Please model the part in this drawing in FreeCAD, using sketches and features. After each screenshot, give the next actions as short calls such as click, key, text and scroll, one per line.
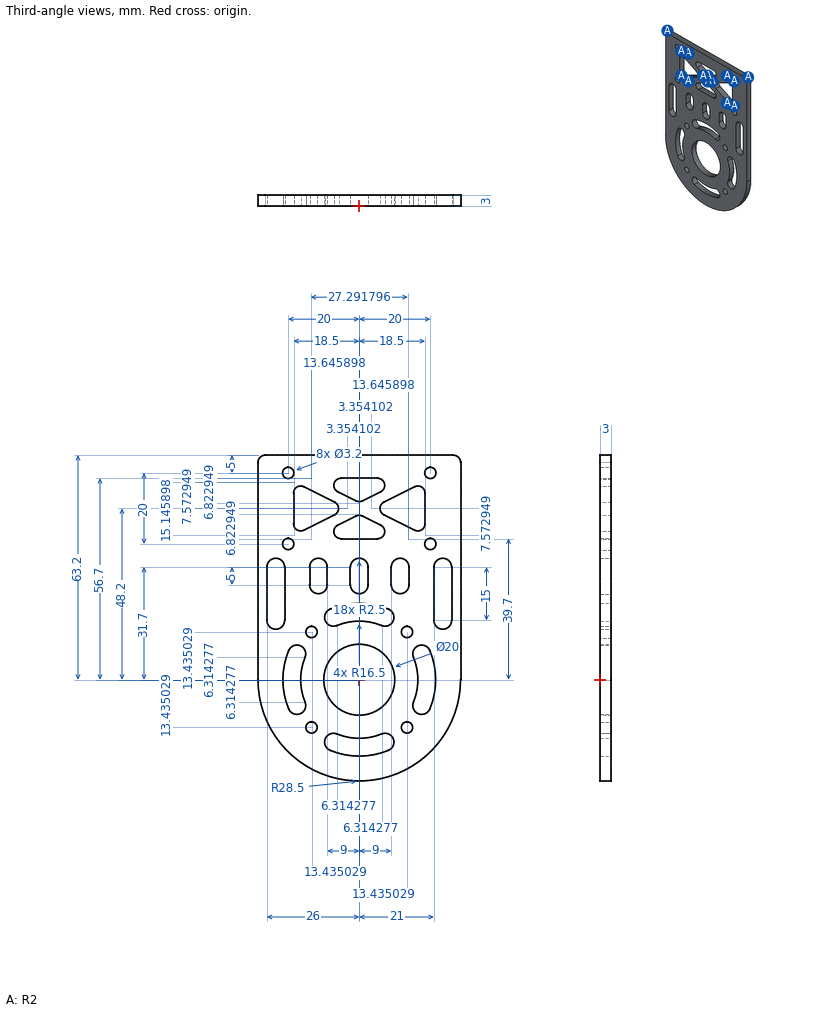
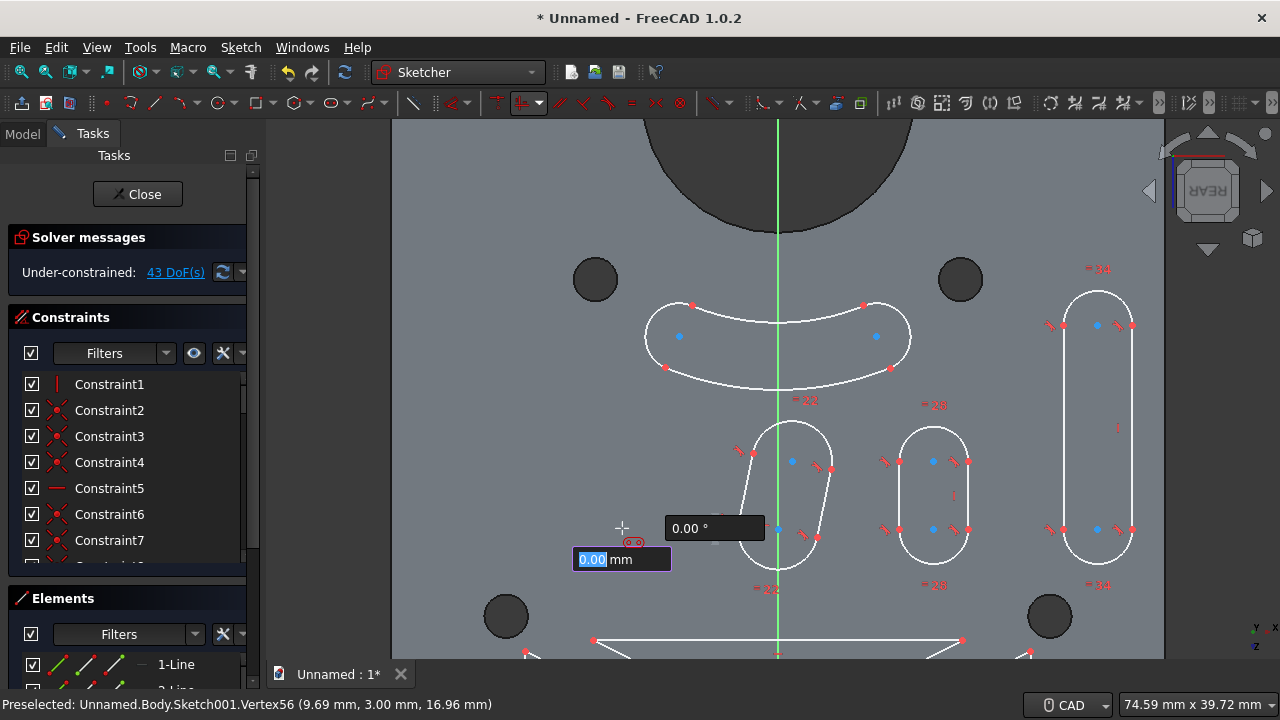
click(622, 460)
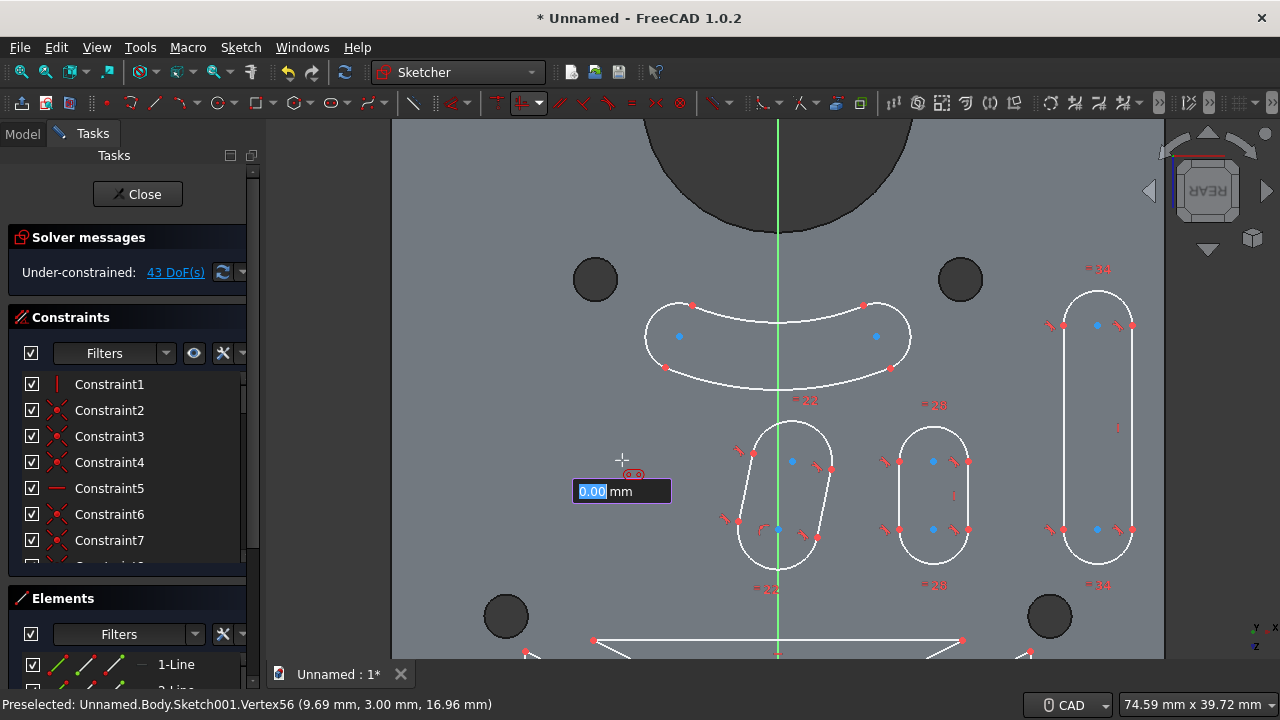
click(588, 494)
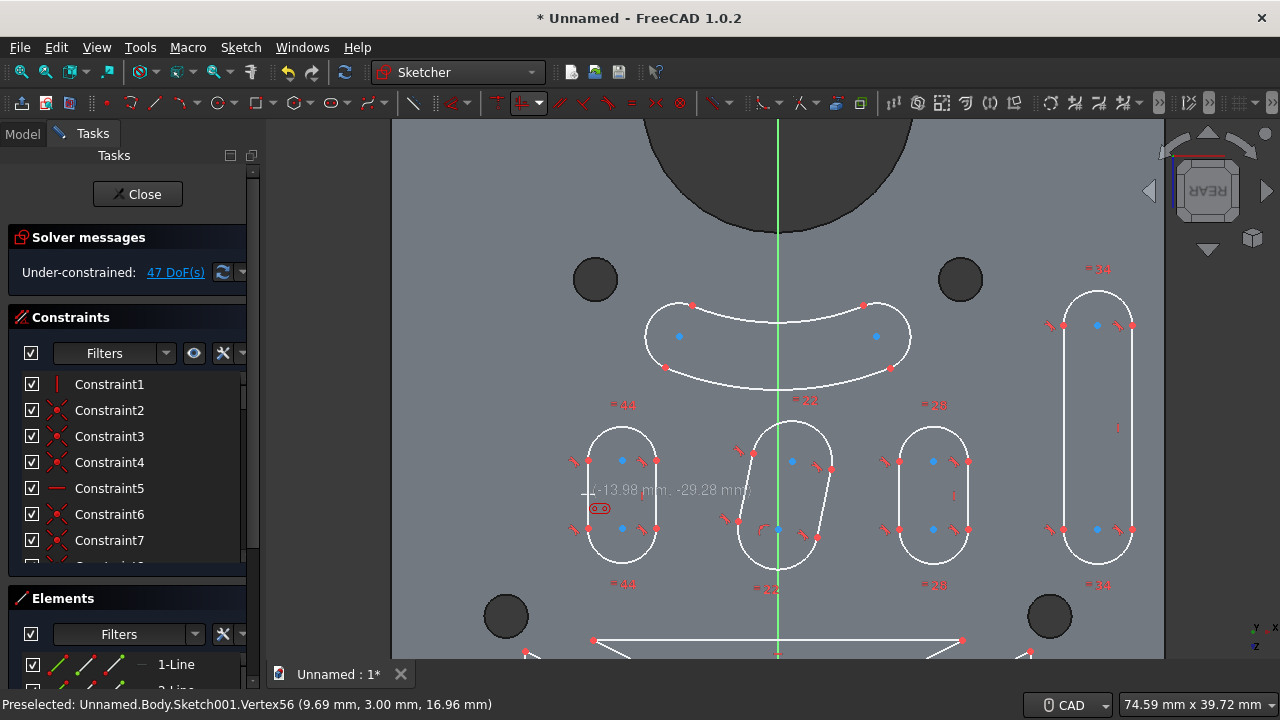
click(459, 528)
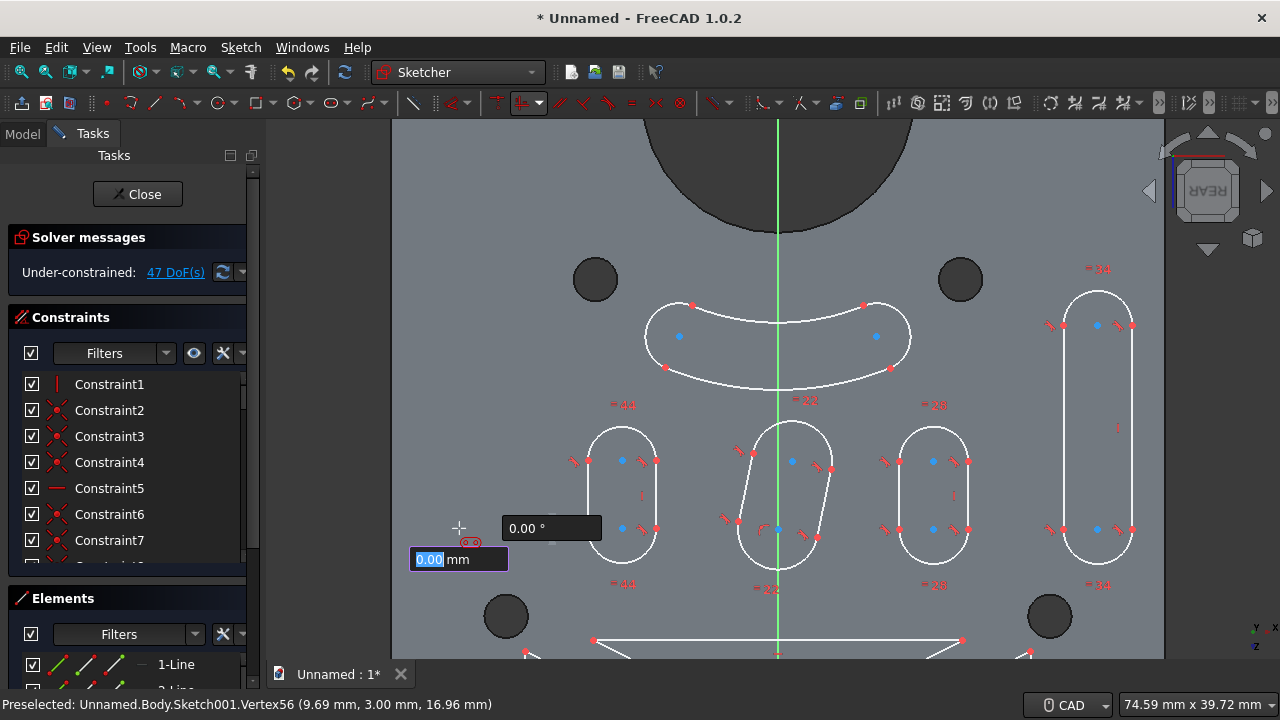
click(459, 324)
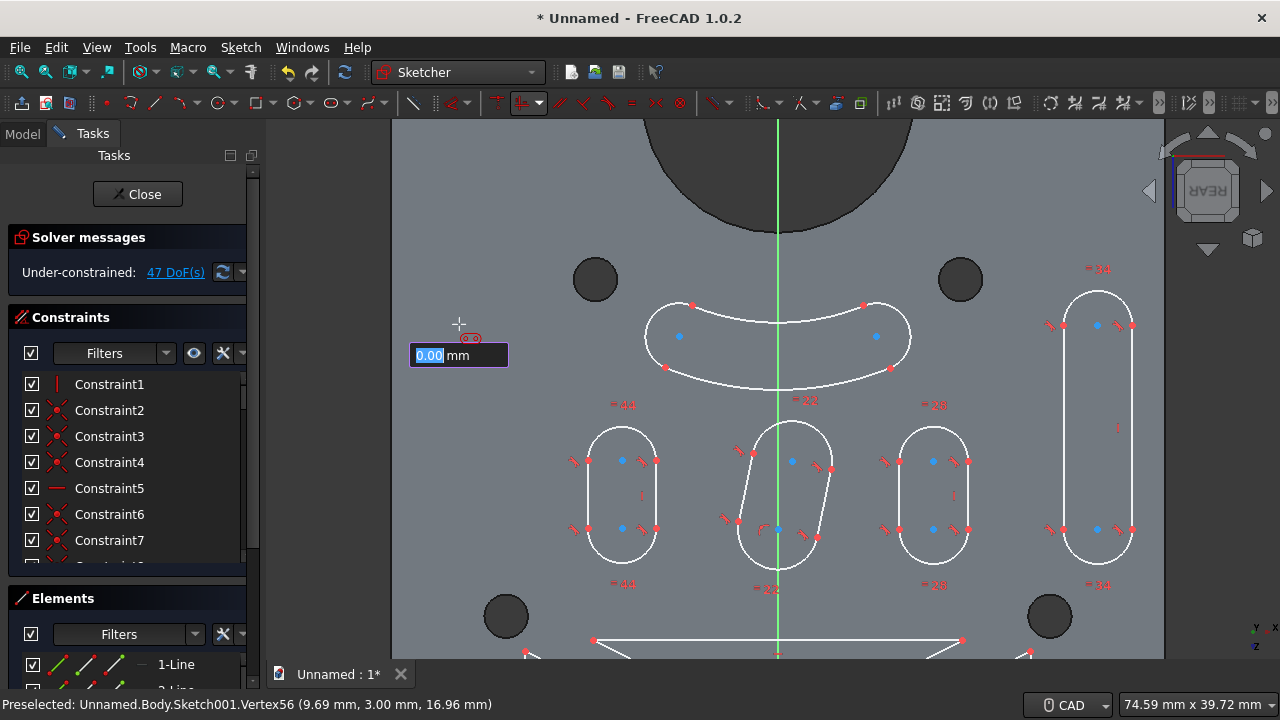
click(425, 426)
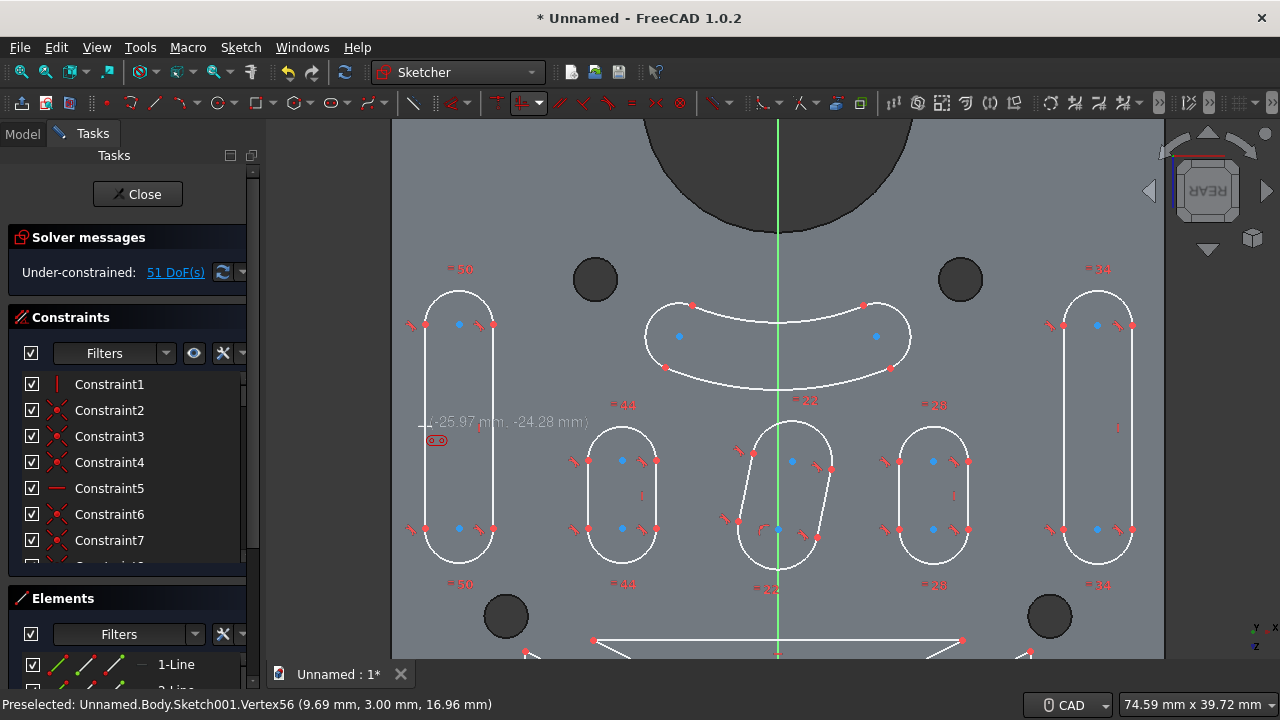
click(180, 104)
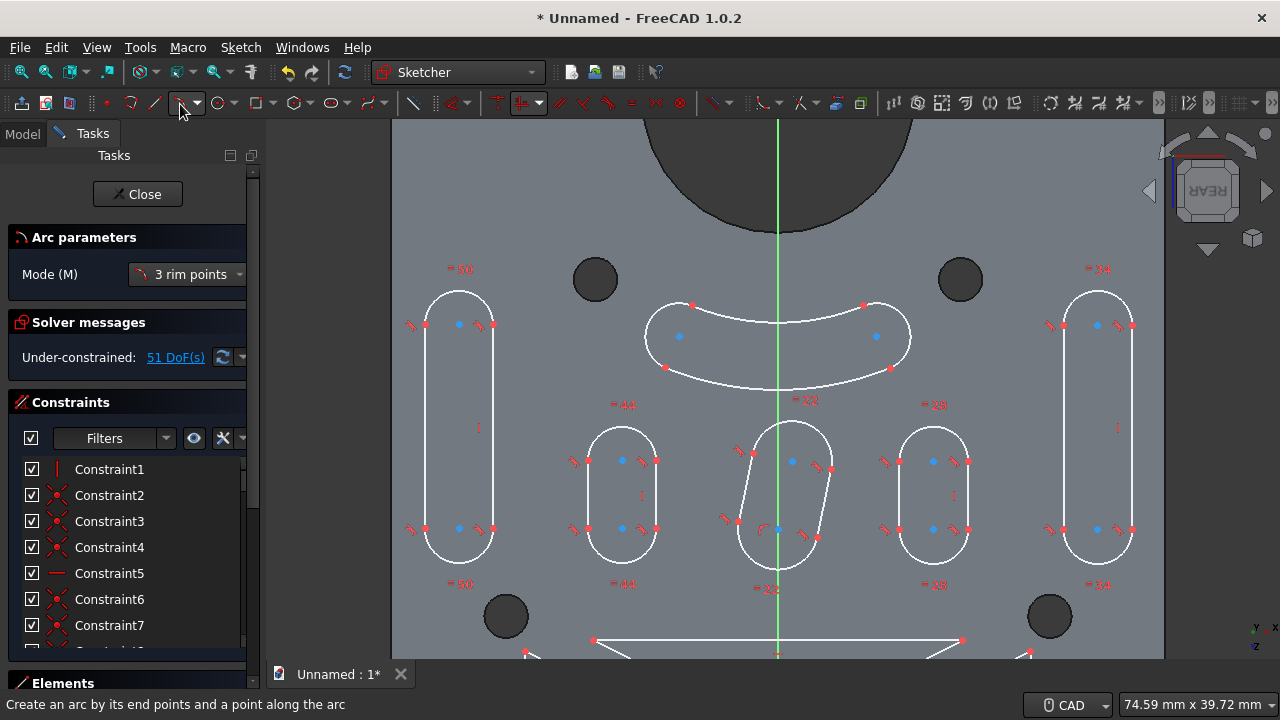
click(571, 183)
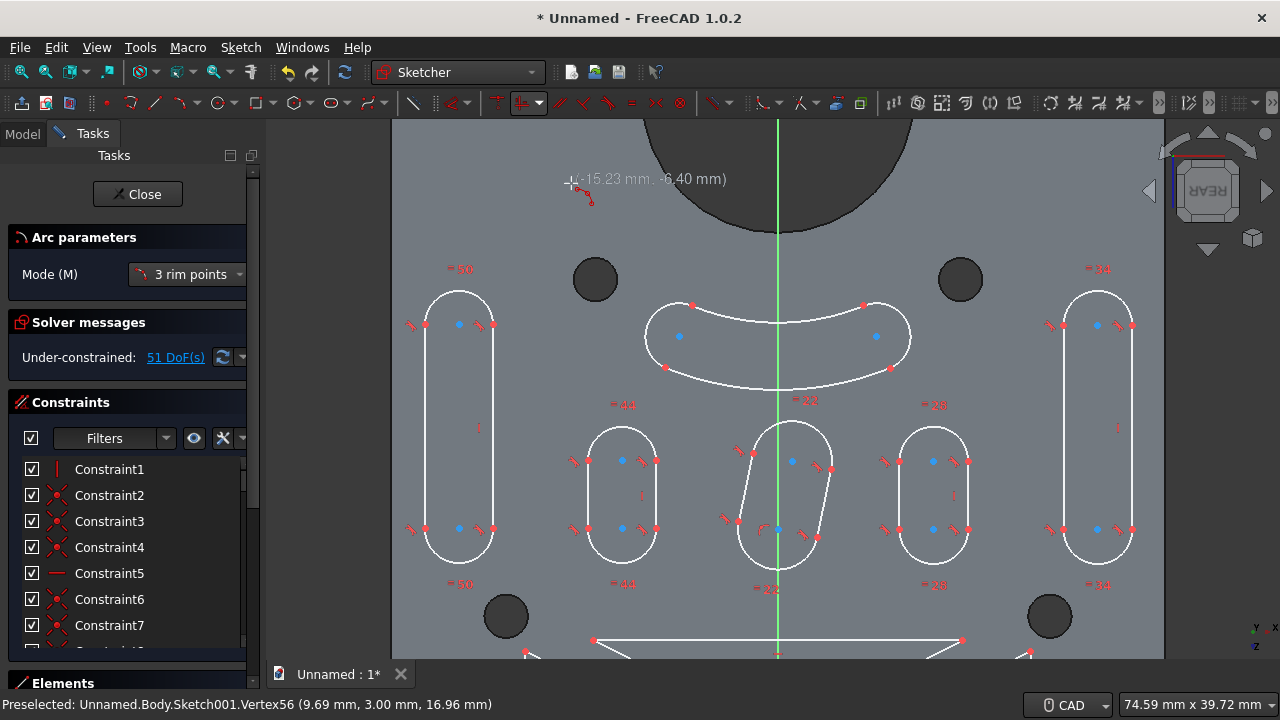
scroll(673, 412, down, 6)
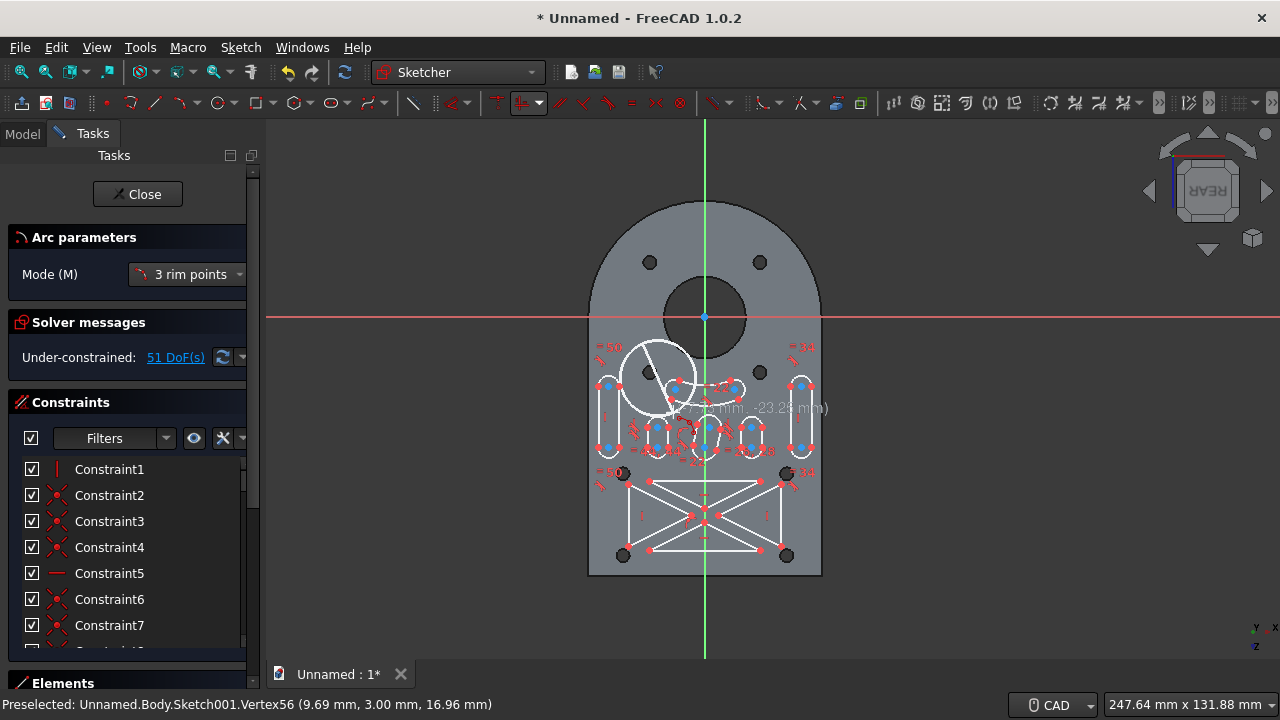
click(643, 292)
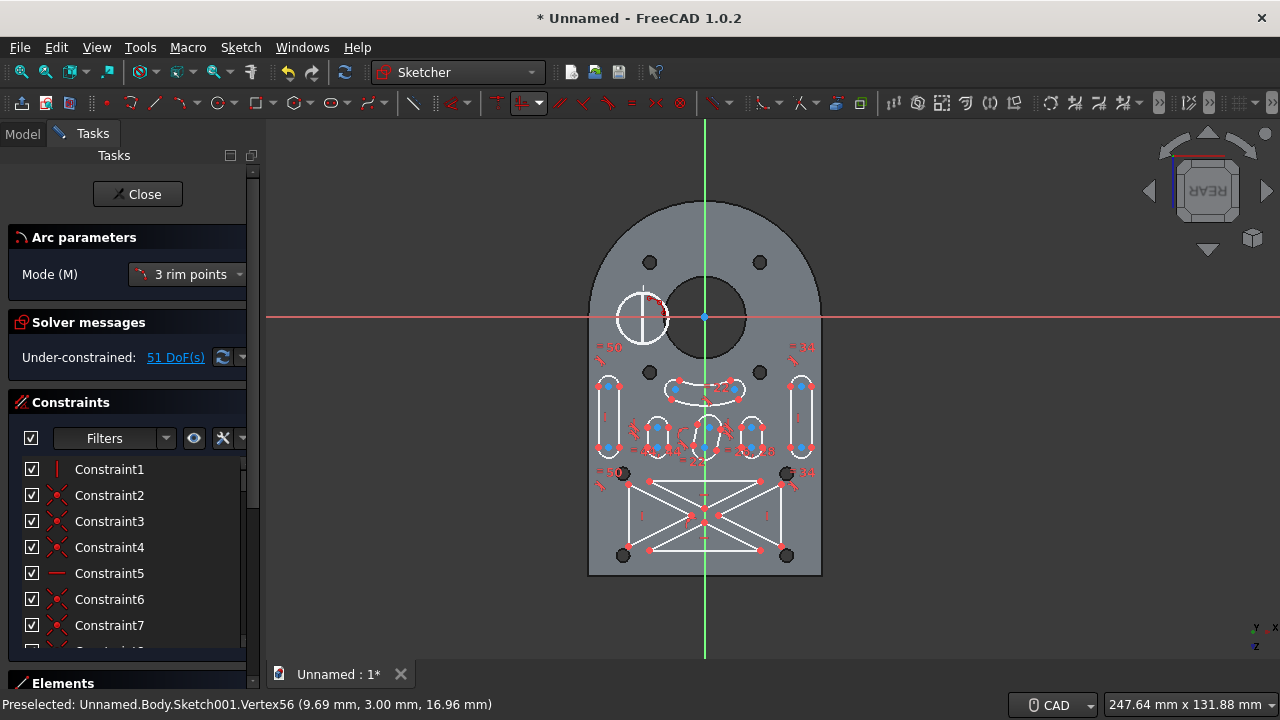
scroll(638, 312, up, 6)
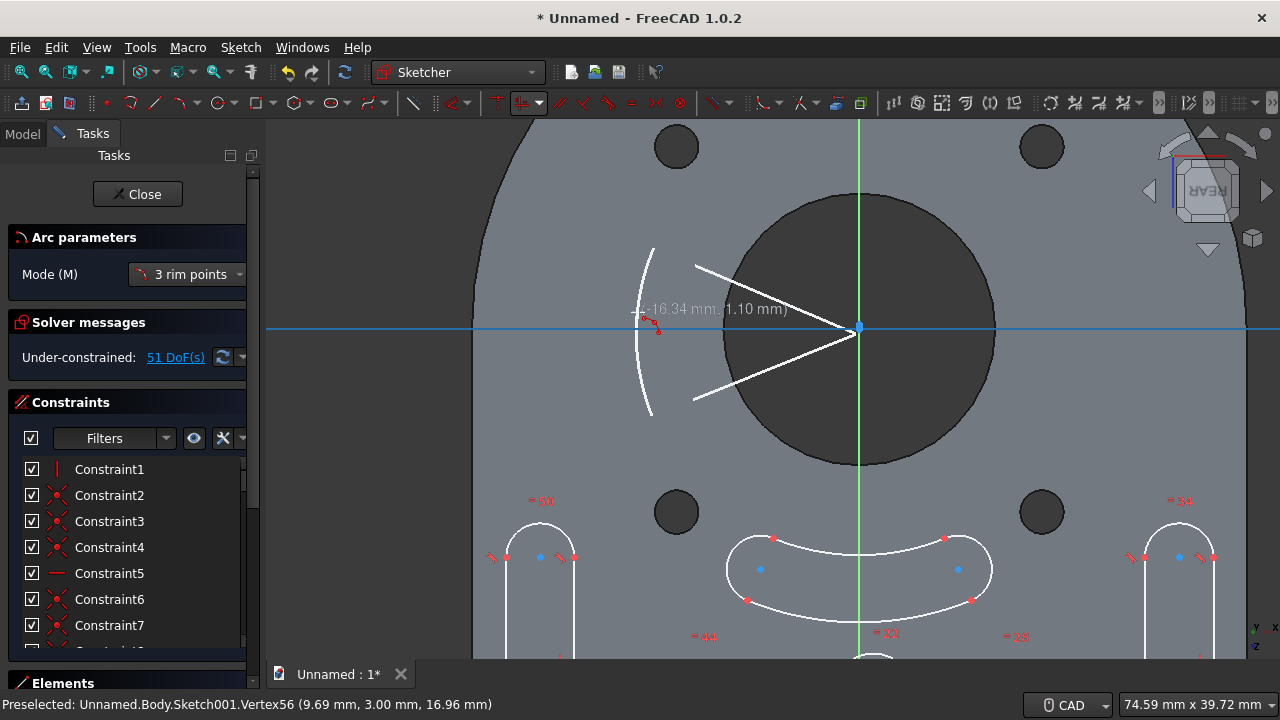
click(636, 312)